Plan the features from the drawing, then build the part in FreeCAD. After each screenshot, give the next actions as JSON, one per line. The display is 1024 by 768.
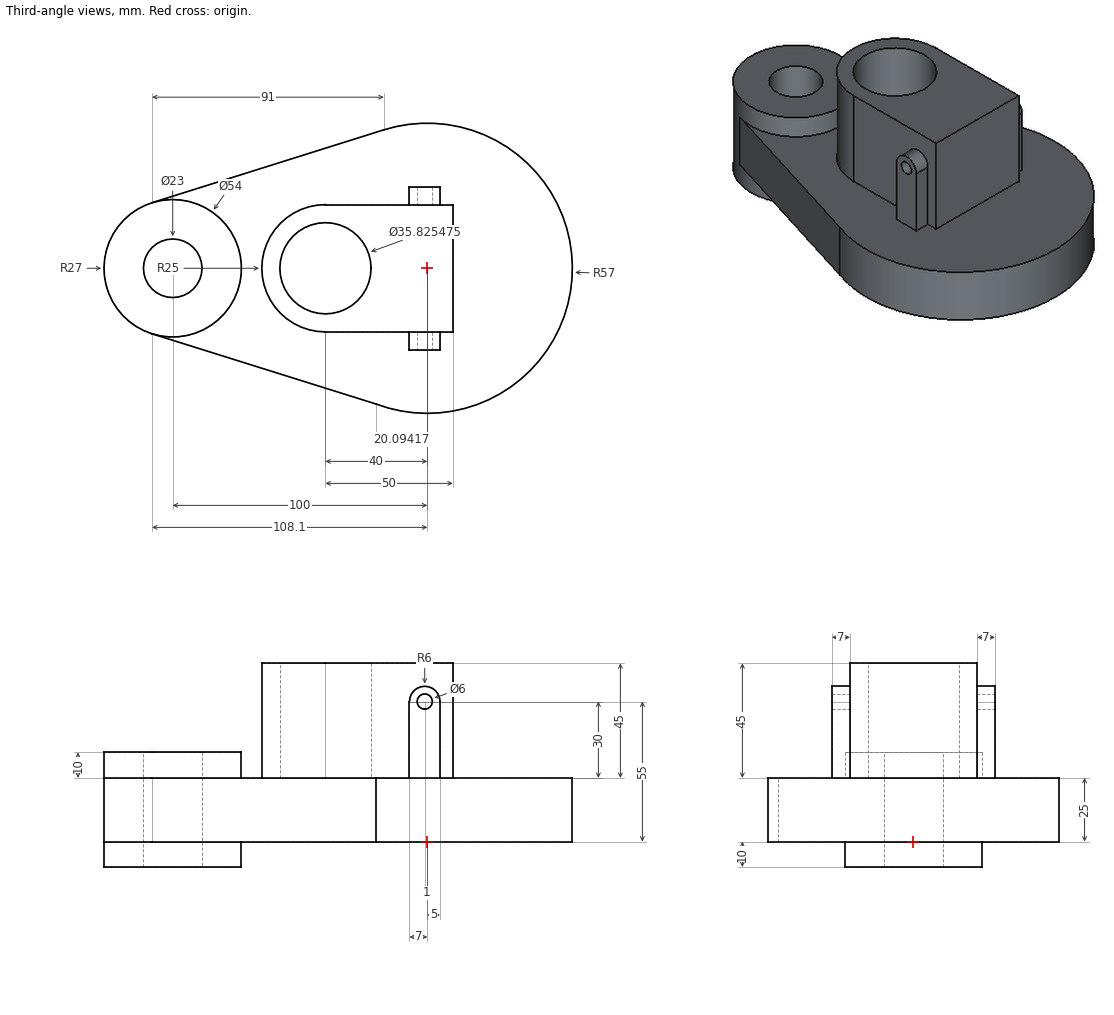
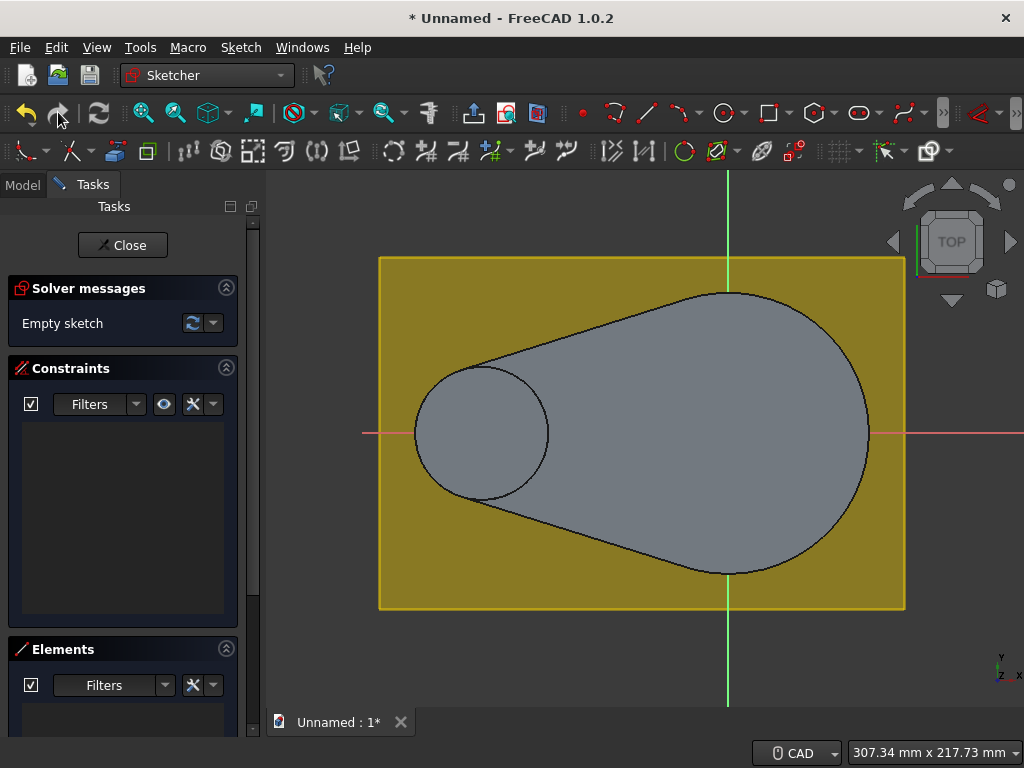
{"action": "left_click", "coordinate": [538, 114]}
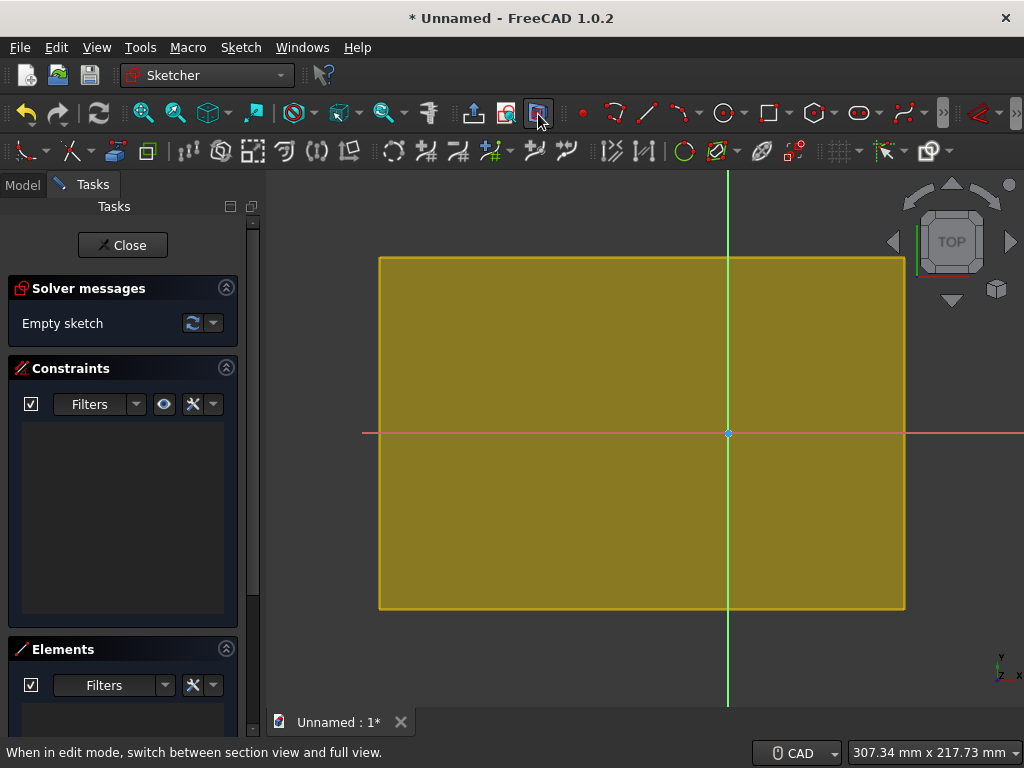
{"action": "key", "text": "g c"}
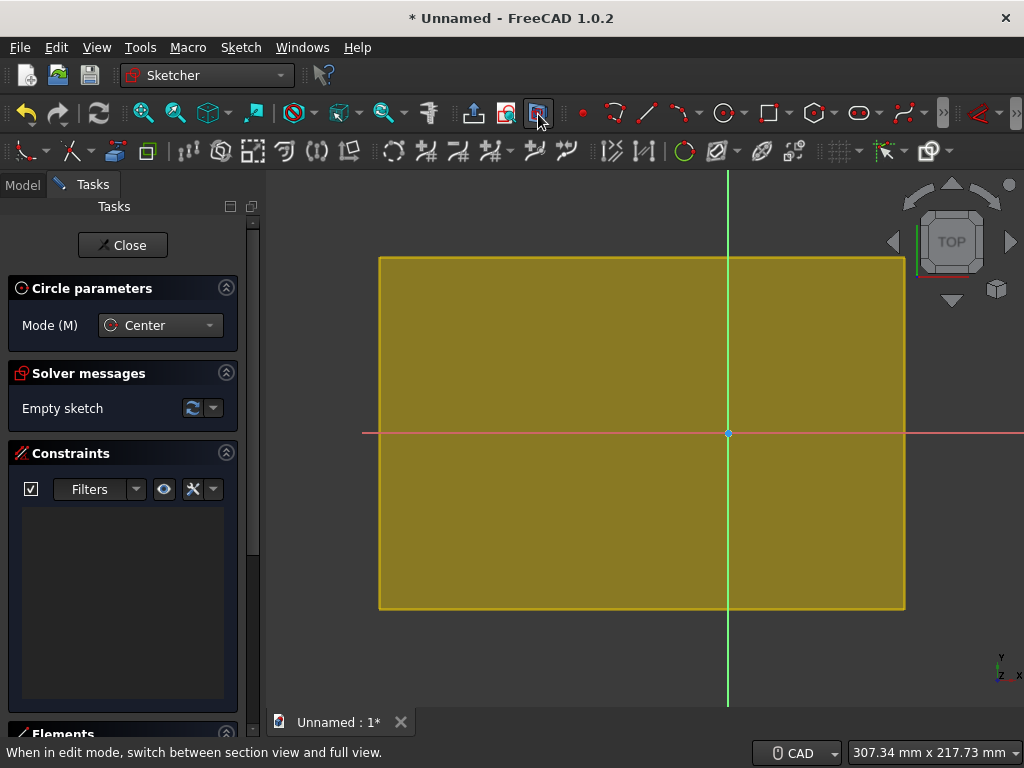
{"action": "left_click", "coordinate": [482, 433]}
{"action": "left_click", "coordinate": [529, 386]}
{"action": "key", "text": "Escape"}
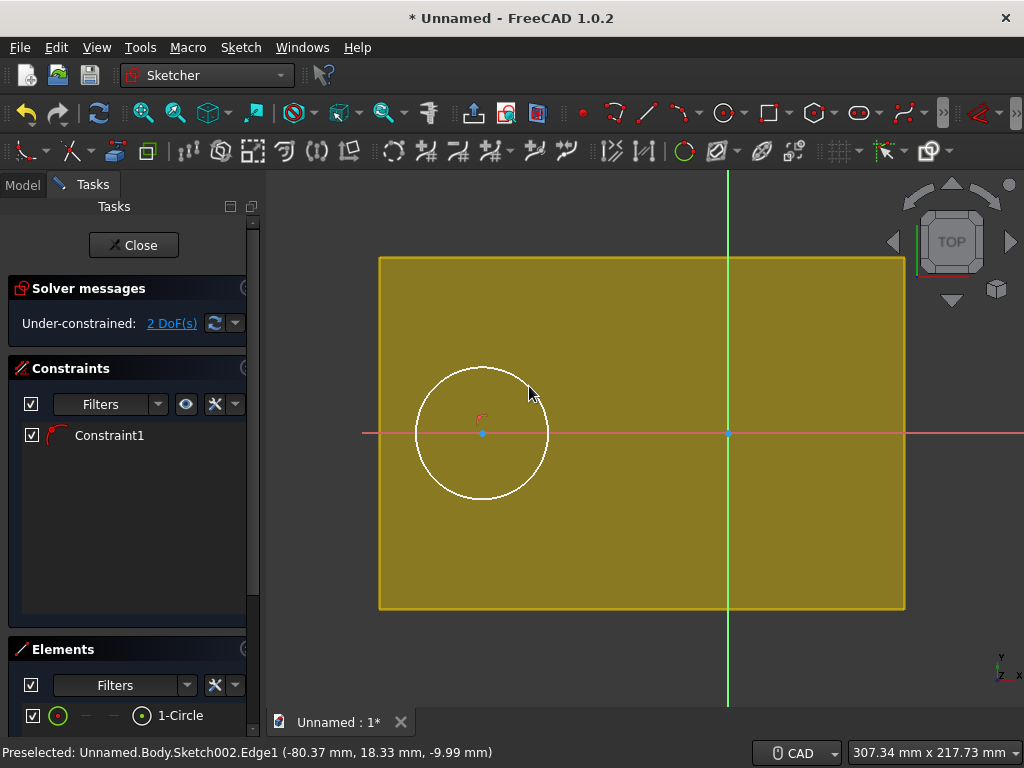
{"action": "key", "text": "d"}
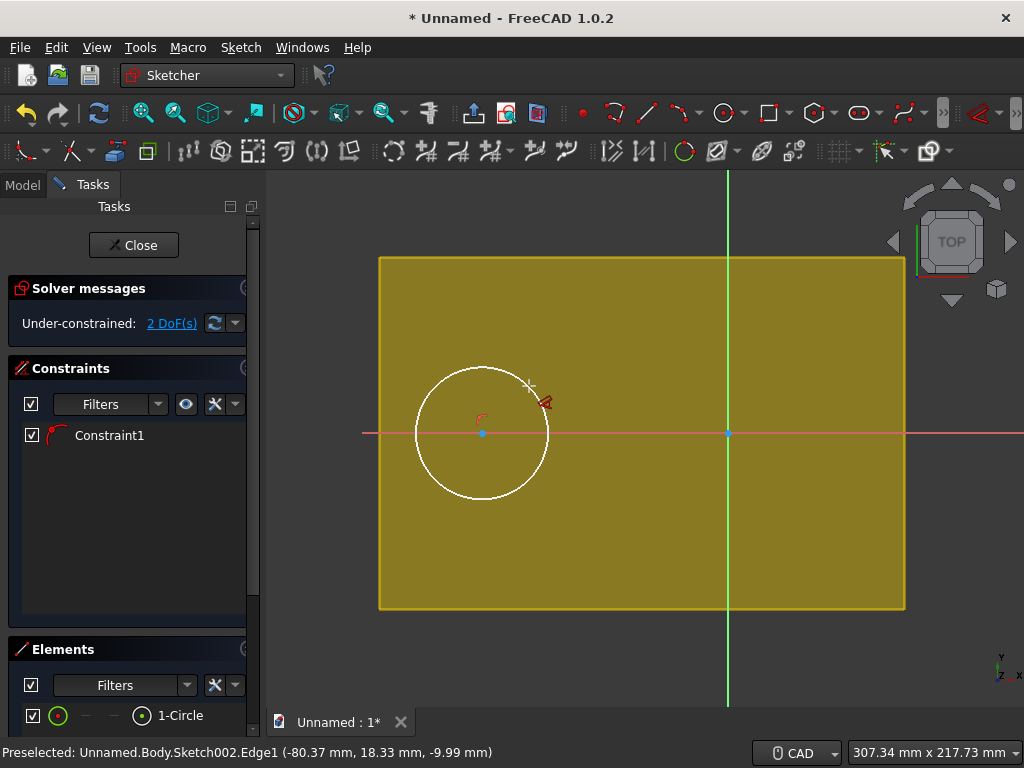
{"action": "left_click", "coordinate": [529, 387]}
{"action": "left_click", "coordinate": [552, 365]}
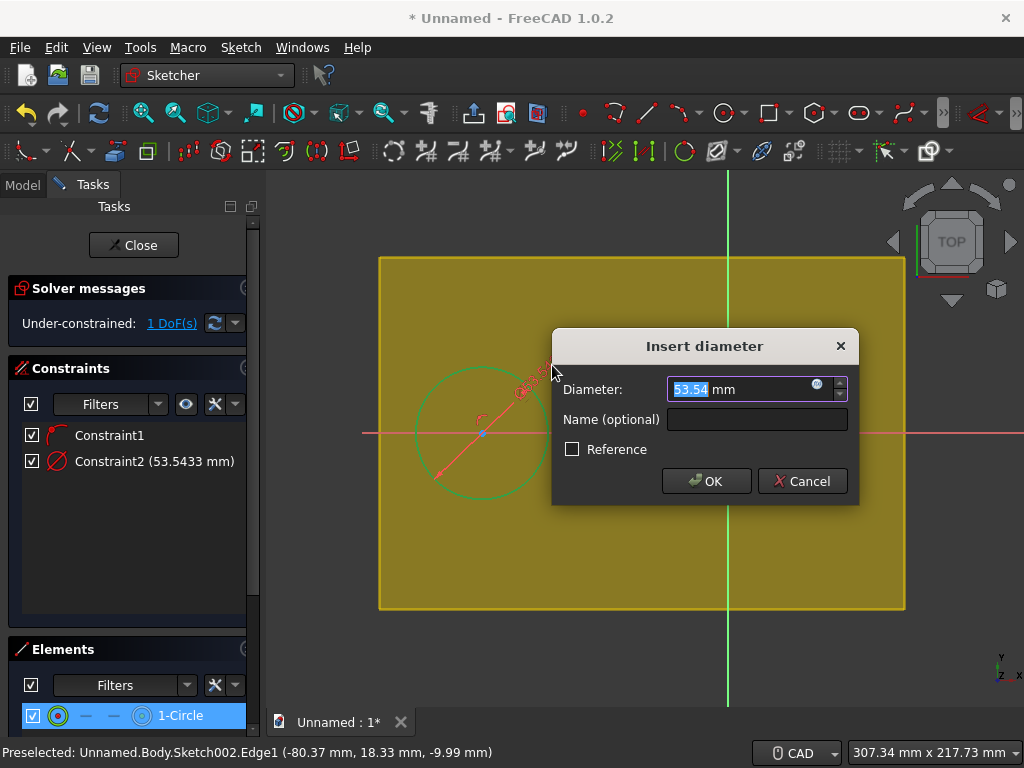
{"action": "type", "text": "54"}
{"action": "key", "text": "Return"}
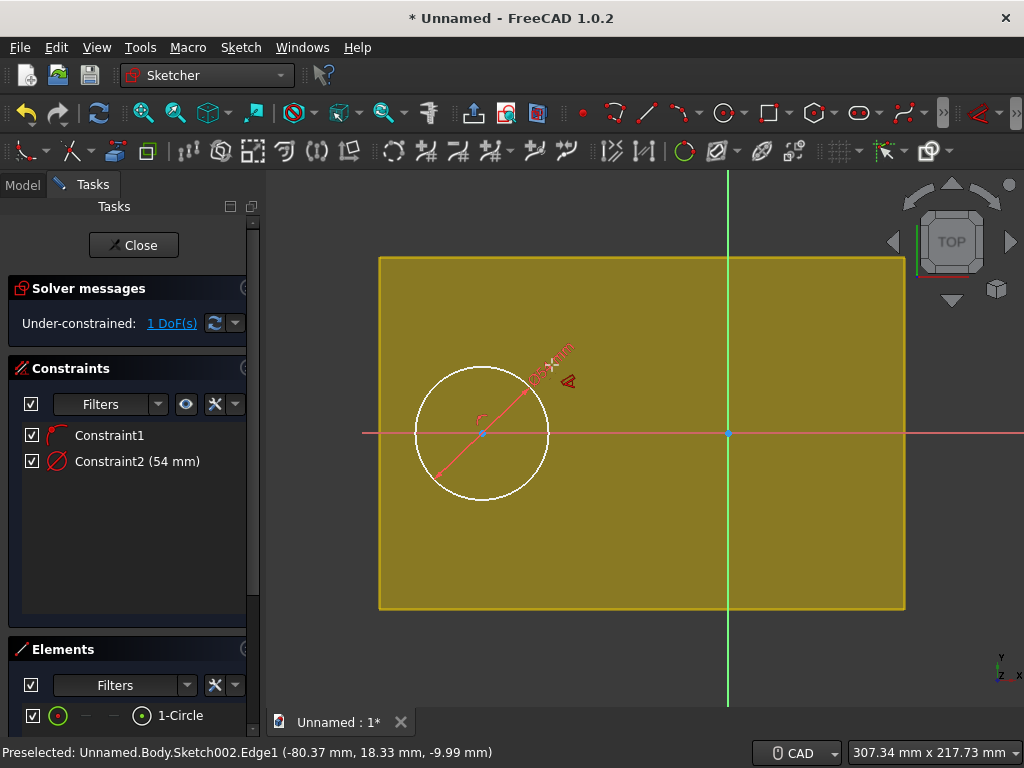
{"action": "left_click", "coordinate": [482, 433]}
{"action": "left_click", "coordinate": [605, 467]}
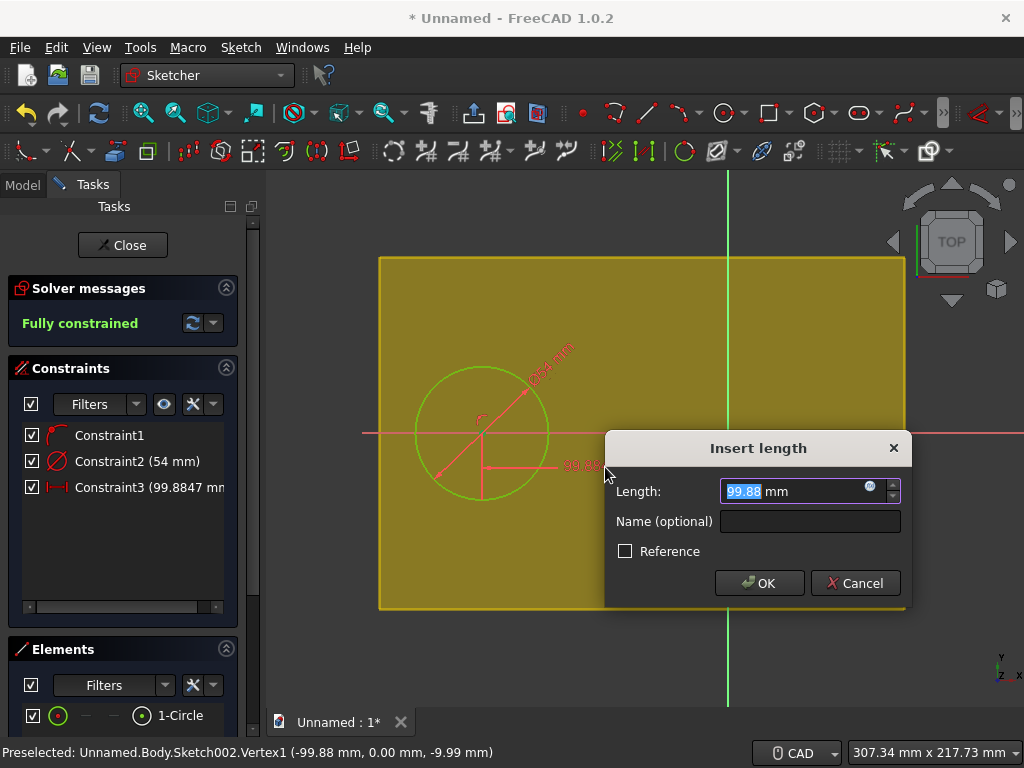
{"action": "type", "text": "100"}
{"action": "key", "text": "Return"}
{"action": "key", "text": "Escape"}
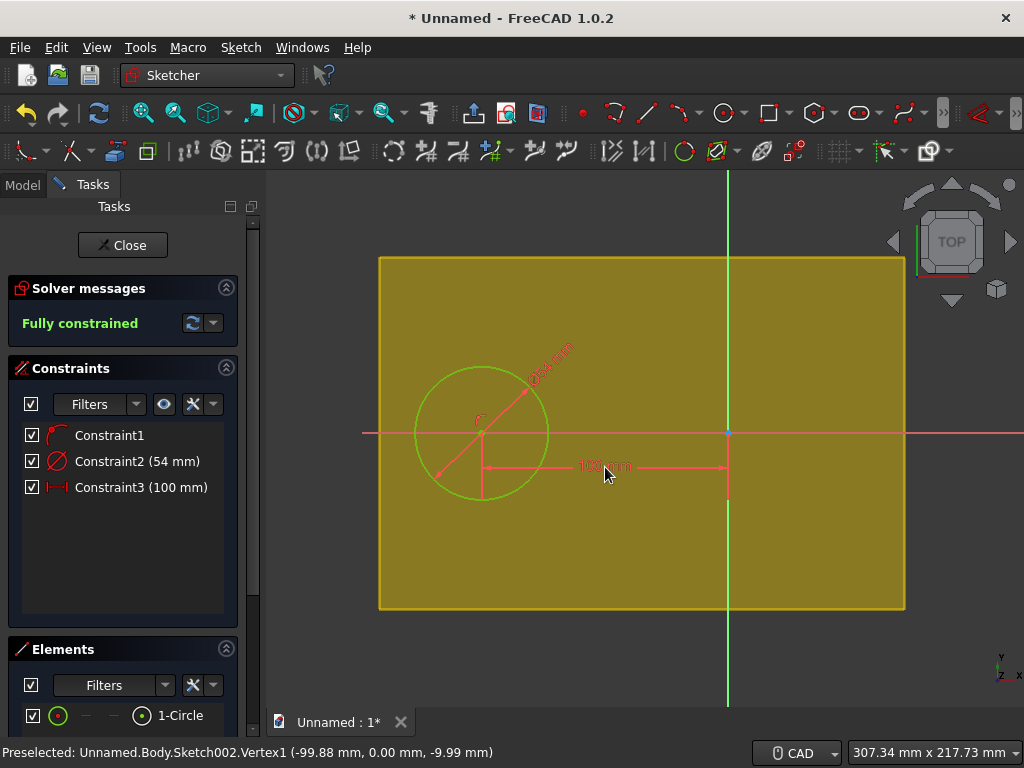
{"action": "left_click", "coordinate": [123, 245]}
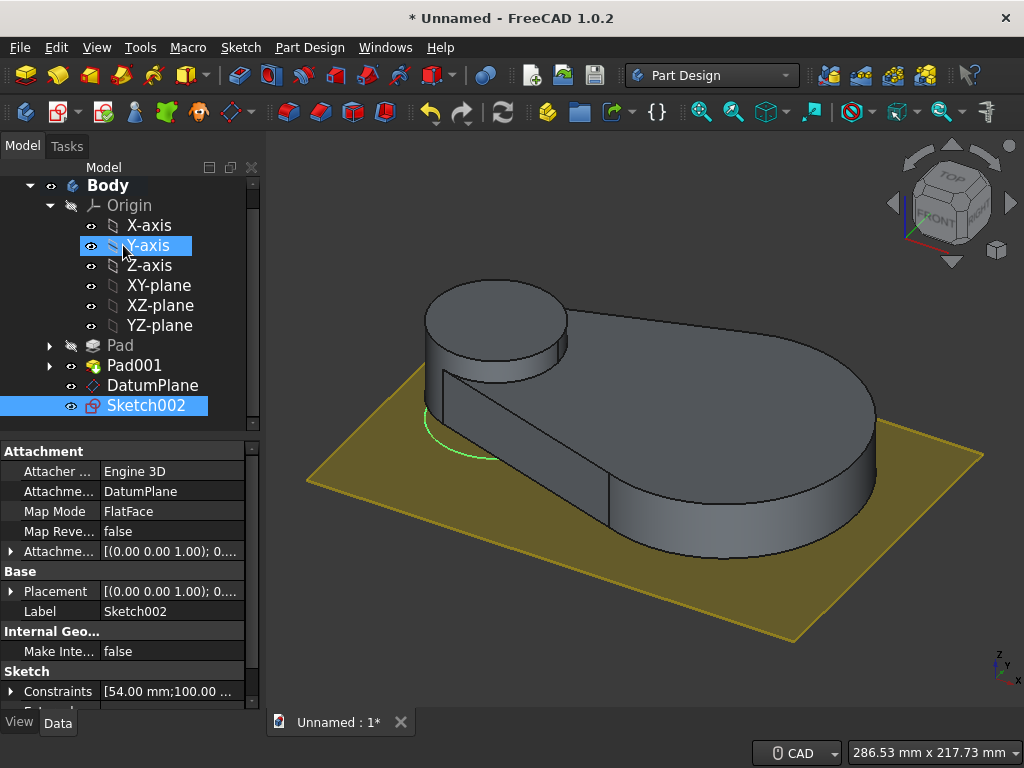
{"action": "left_click", "coordinate": [26, 76]}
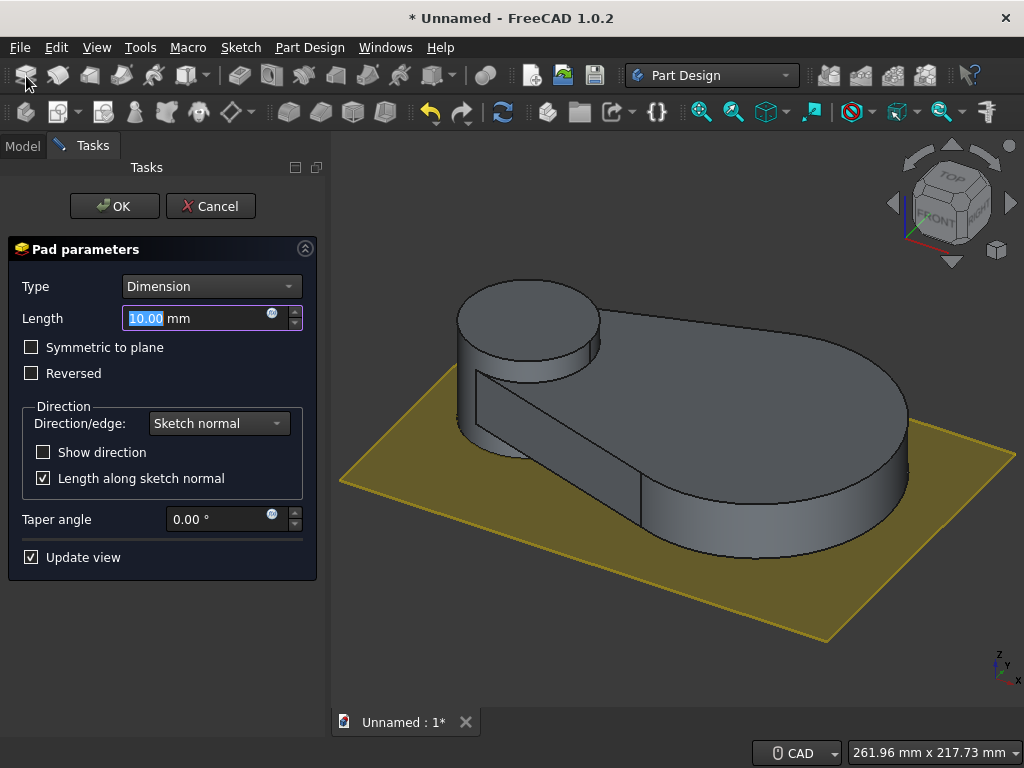
{"action": "type", "text": "10"}
{"action": "key", "text": "Tab"}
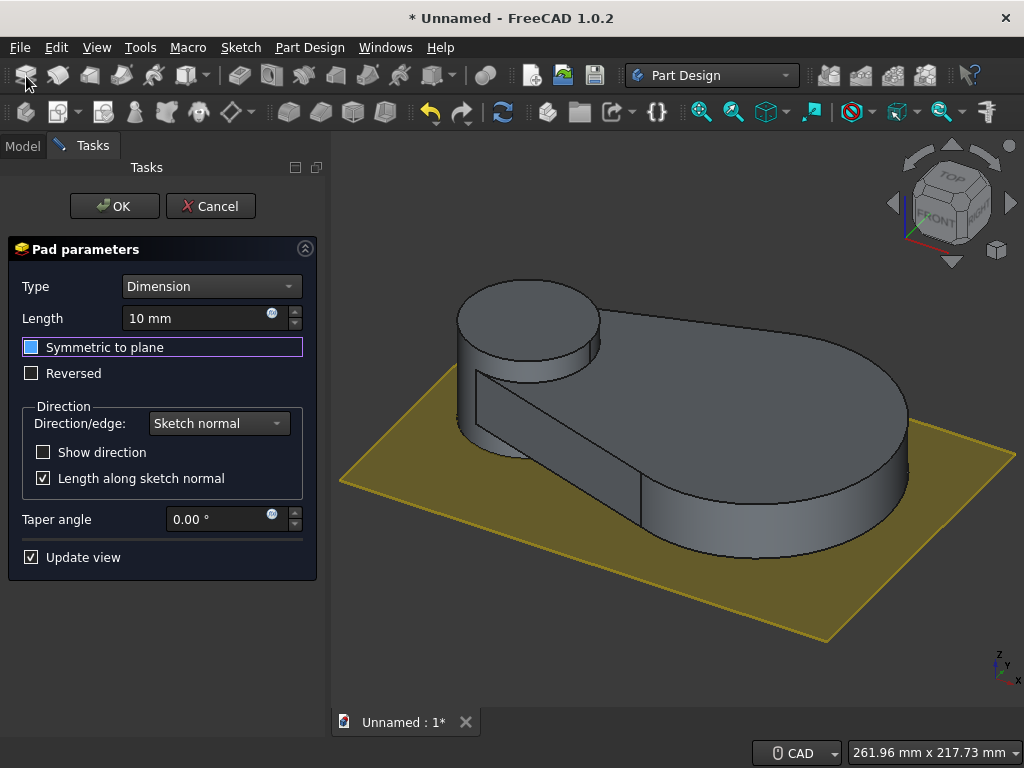
{"action": "left_click", "coordinate": [115, 206]}